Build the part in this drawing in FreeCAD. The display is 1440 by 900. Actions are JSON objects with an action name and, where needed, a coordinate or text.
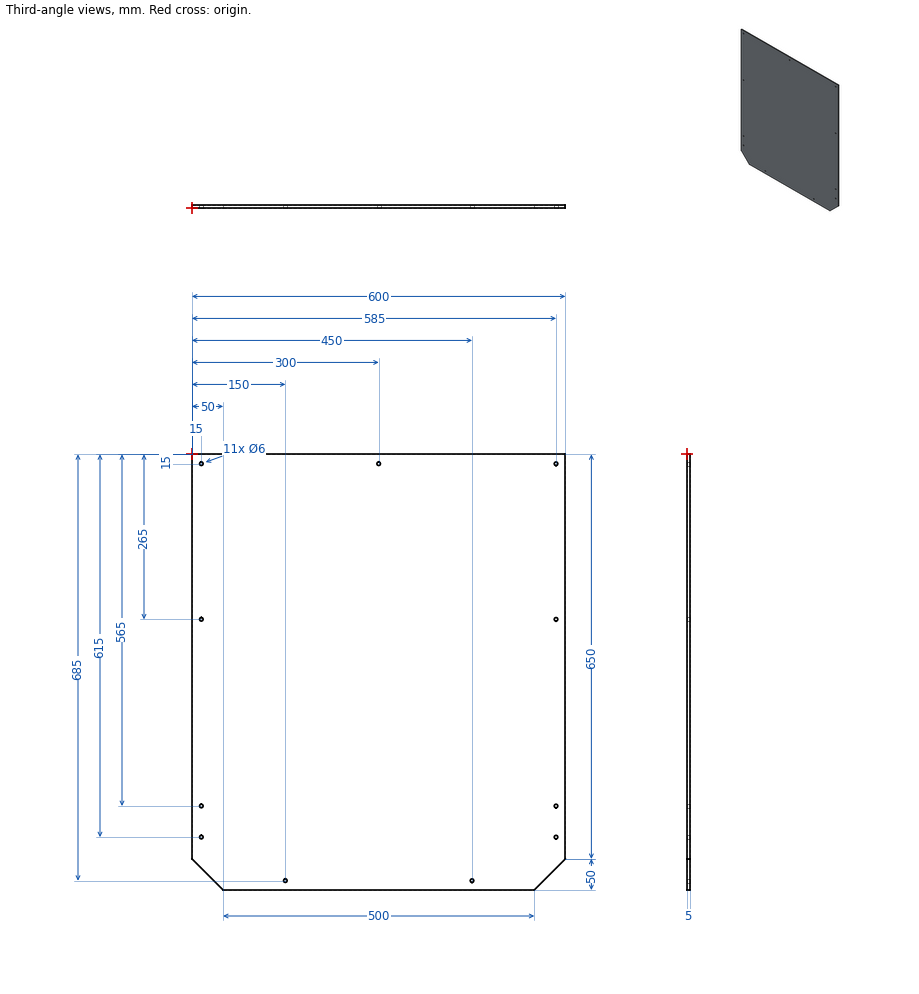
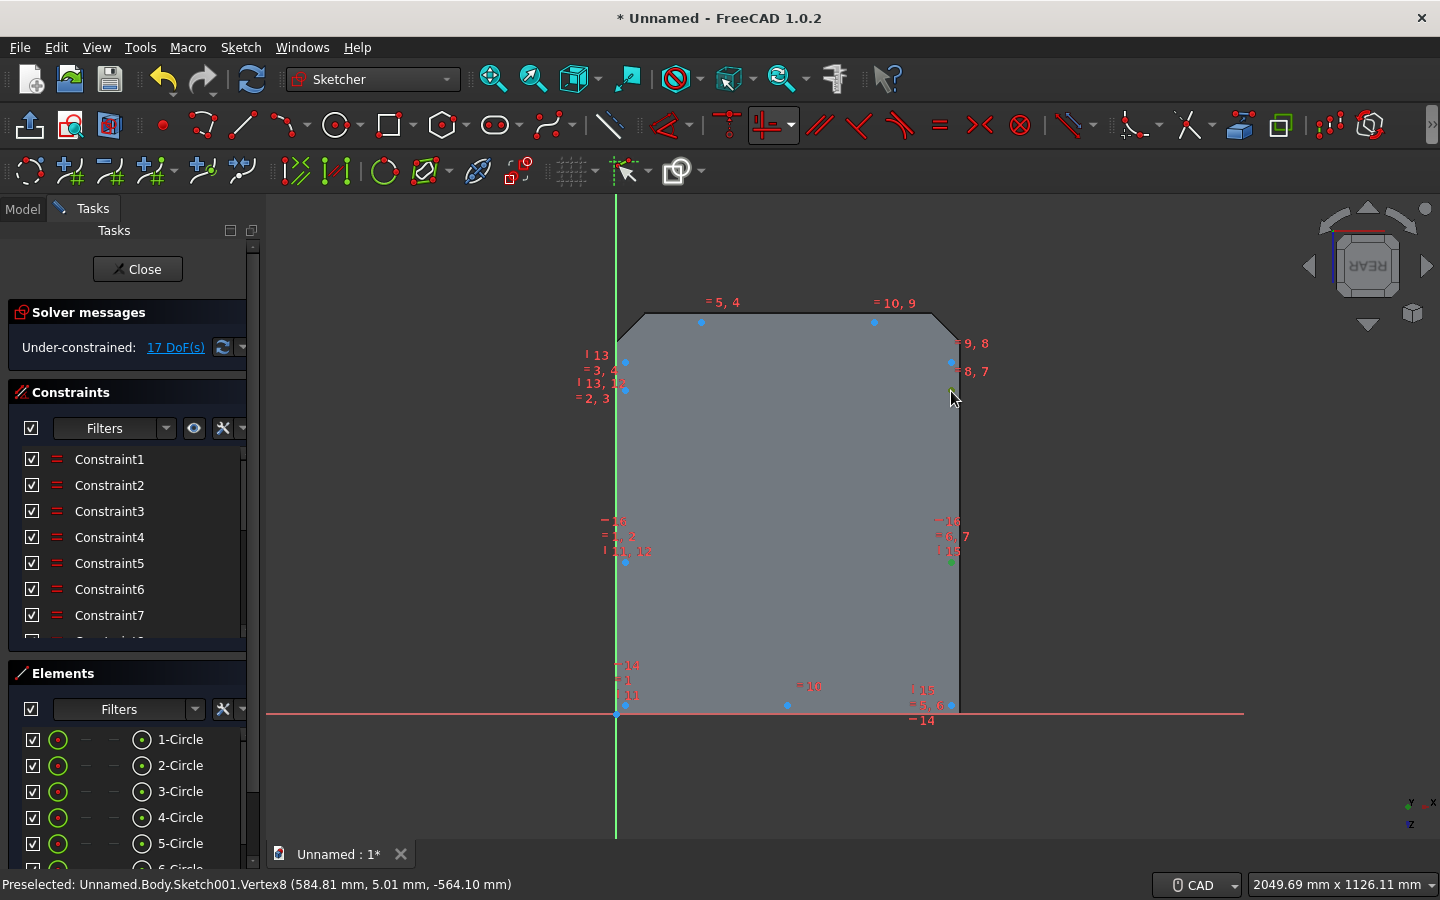
{"action": "key", "text": "v"}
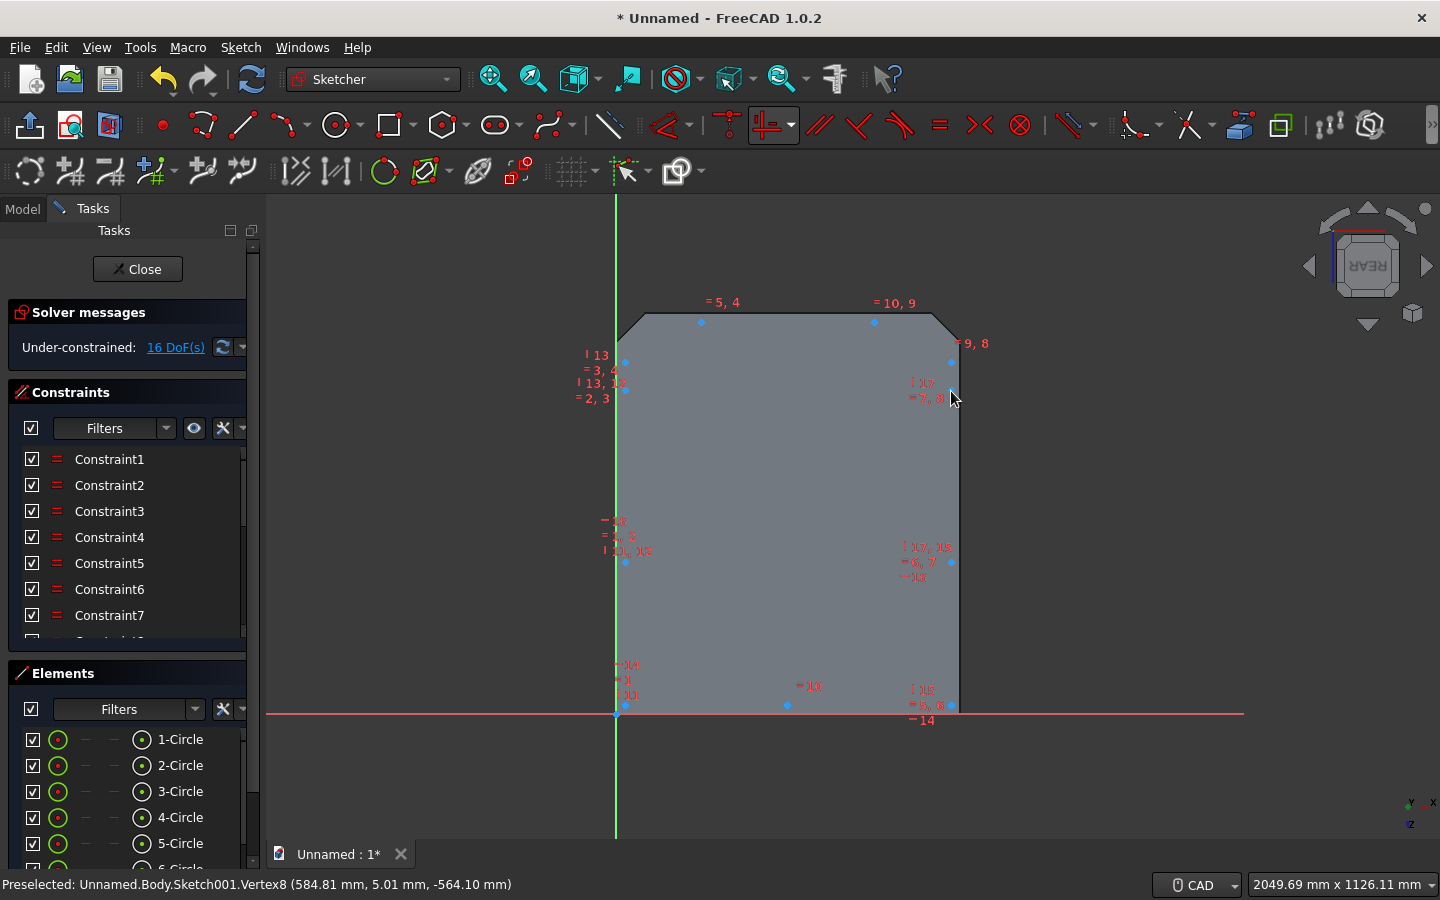
{"action": "left_click", "coordinate": [625, 391]}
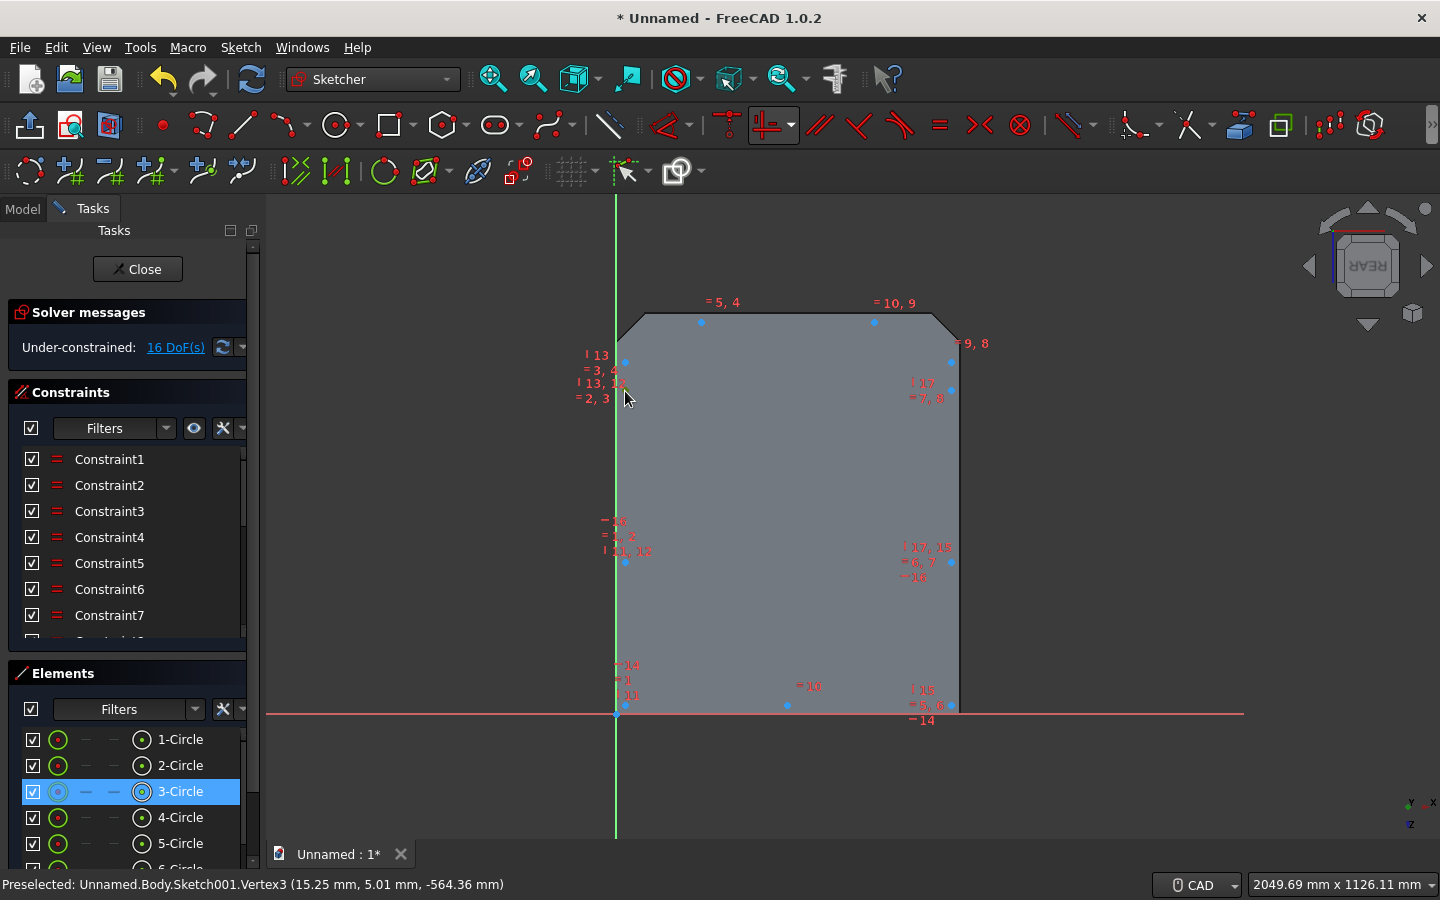
{"action": "left_click", "coordinate": [951, 391]}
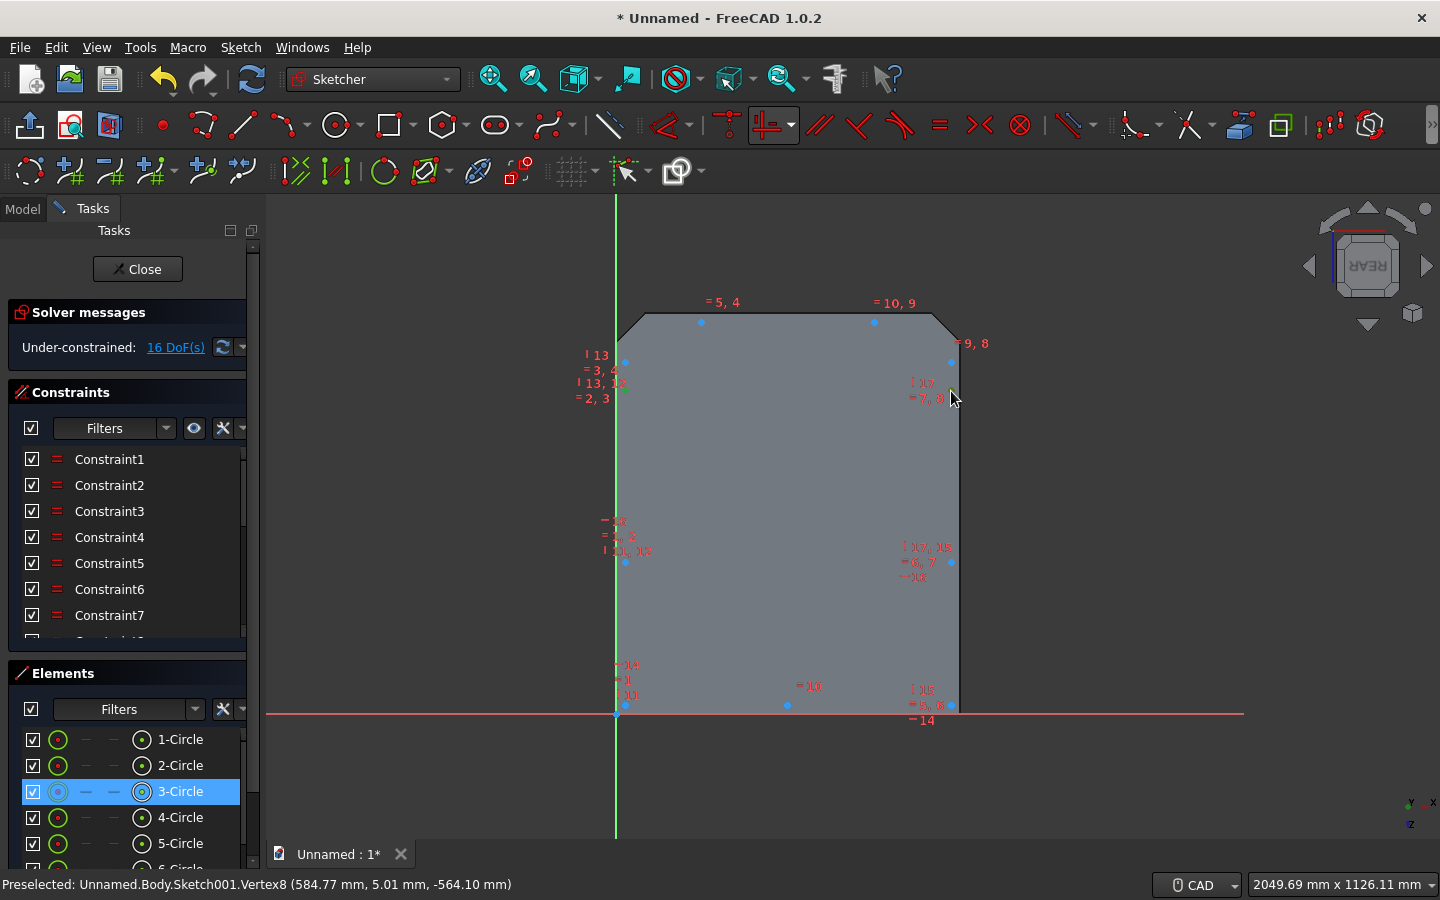
{"action": "key", "text": "h"}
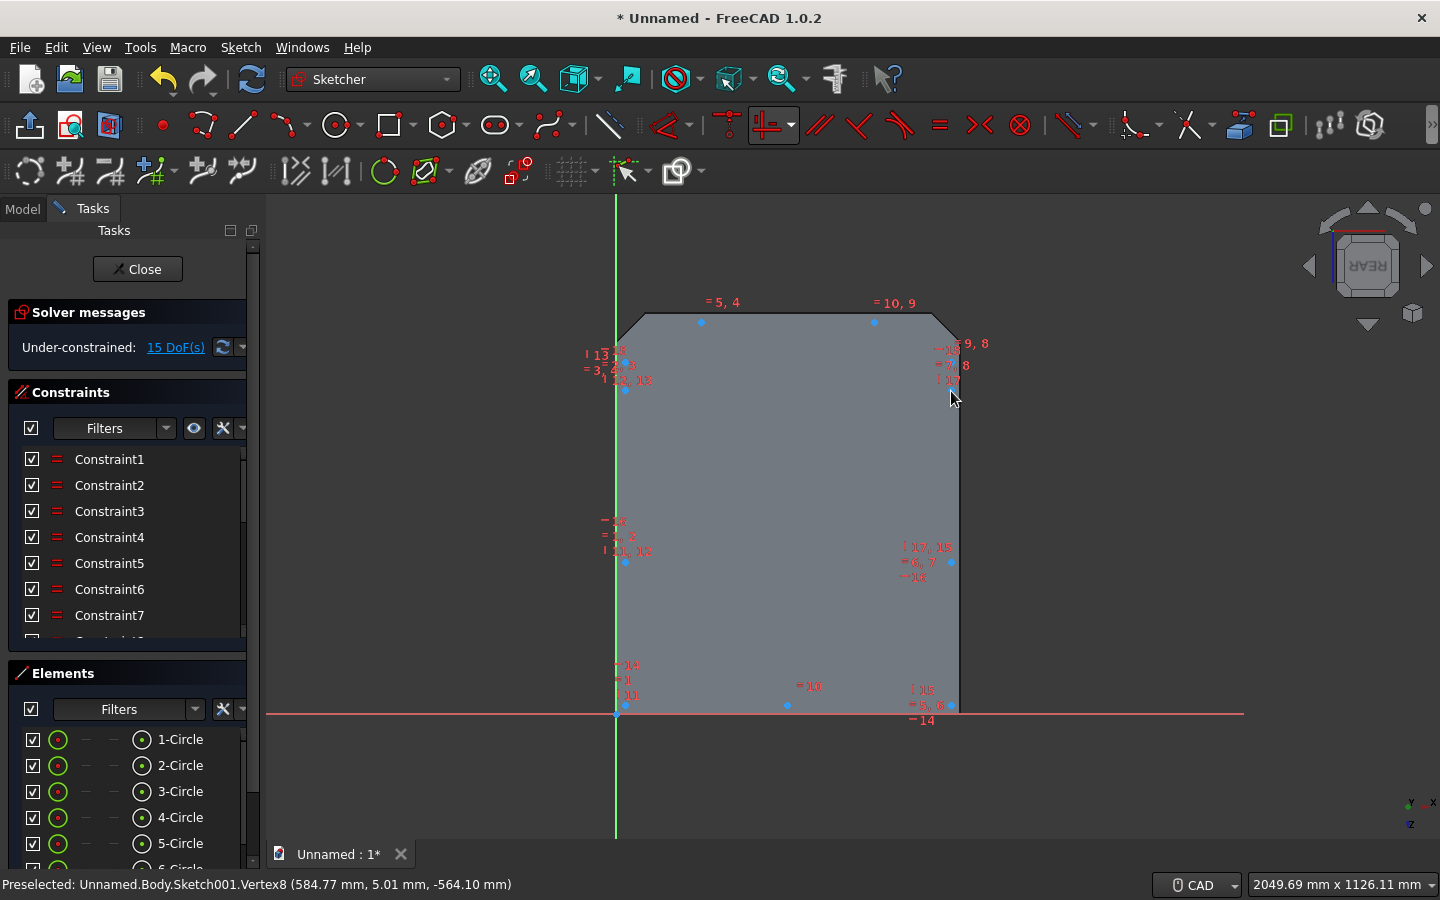
{"action": "left_click", "coordinate": [951, 391]}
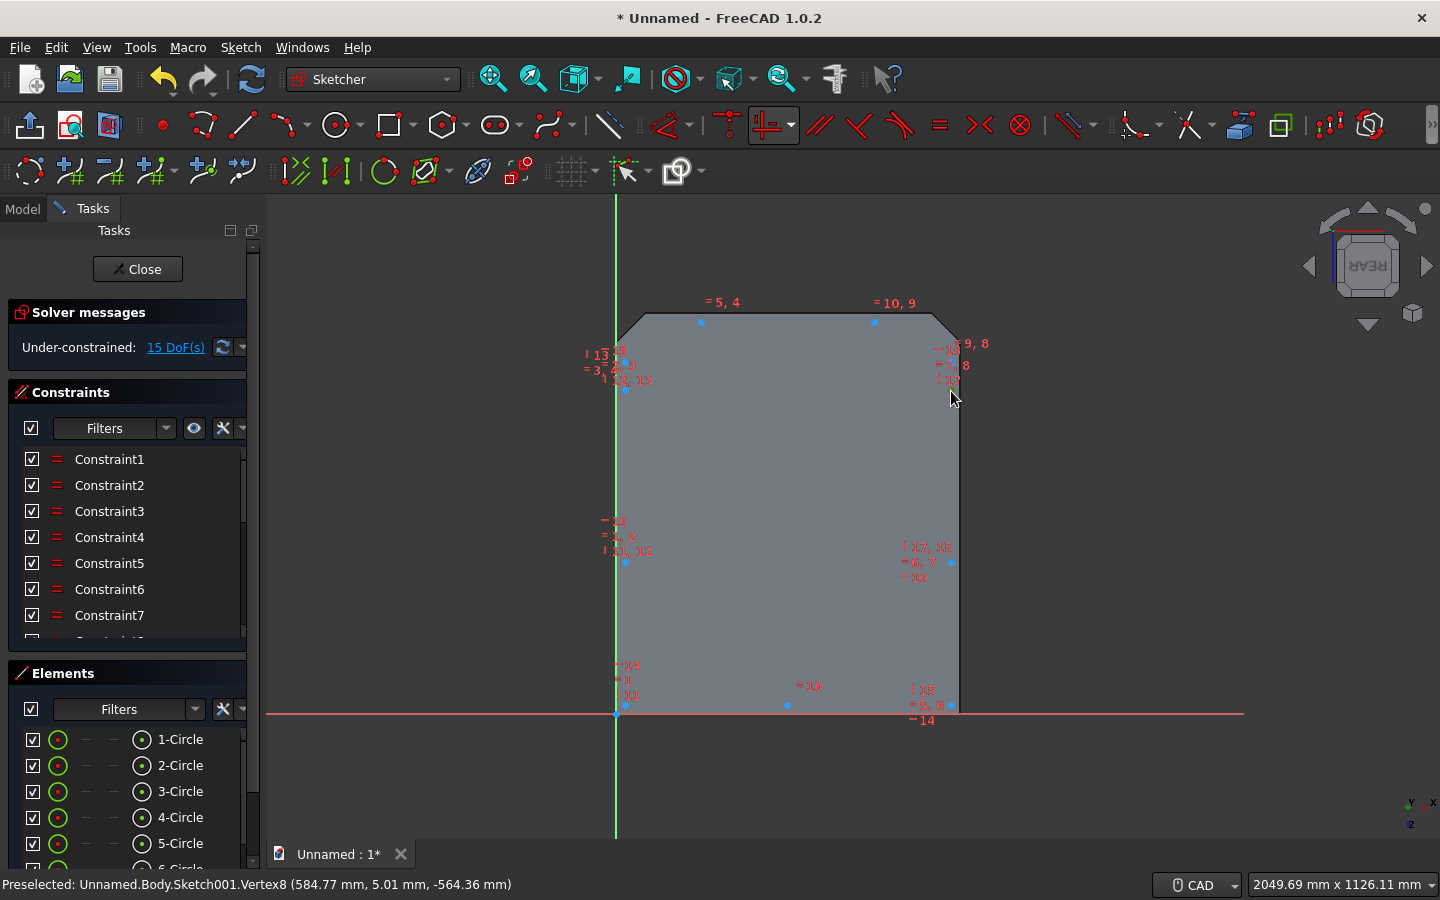
{"action": "scroll", "coordinate": [951, 363], "scroll_direction": "up", "scroll_amount": 4}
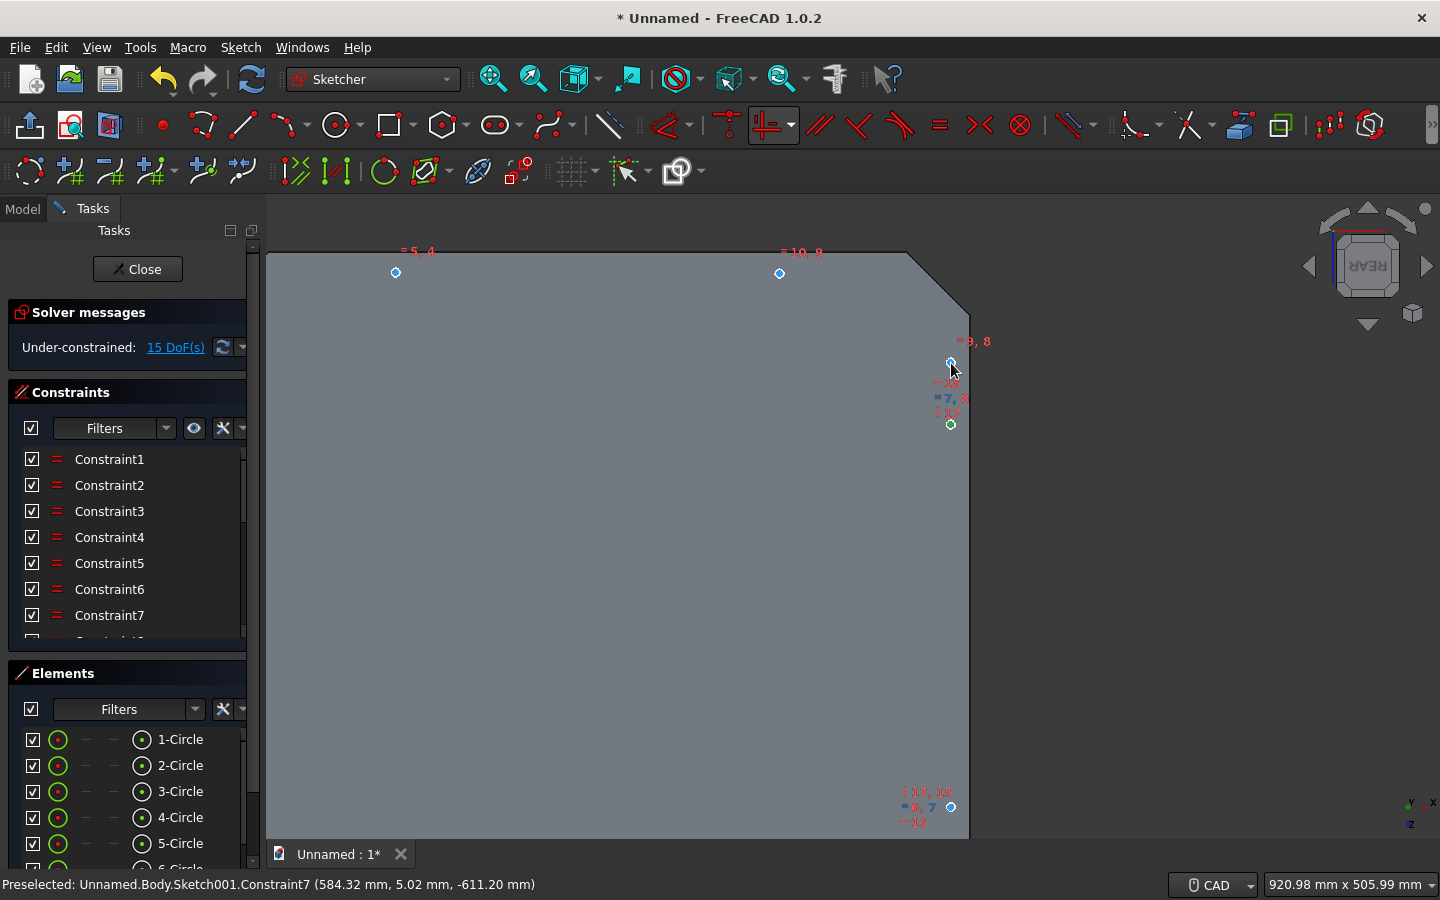
{"action": "left_click", "coordinate": [951, 363]}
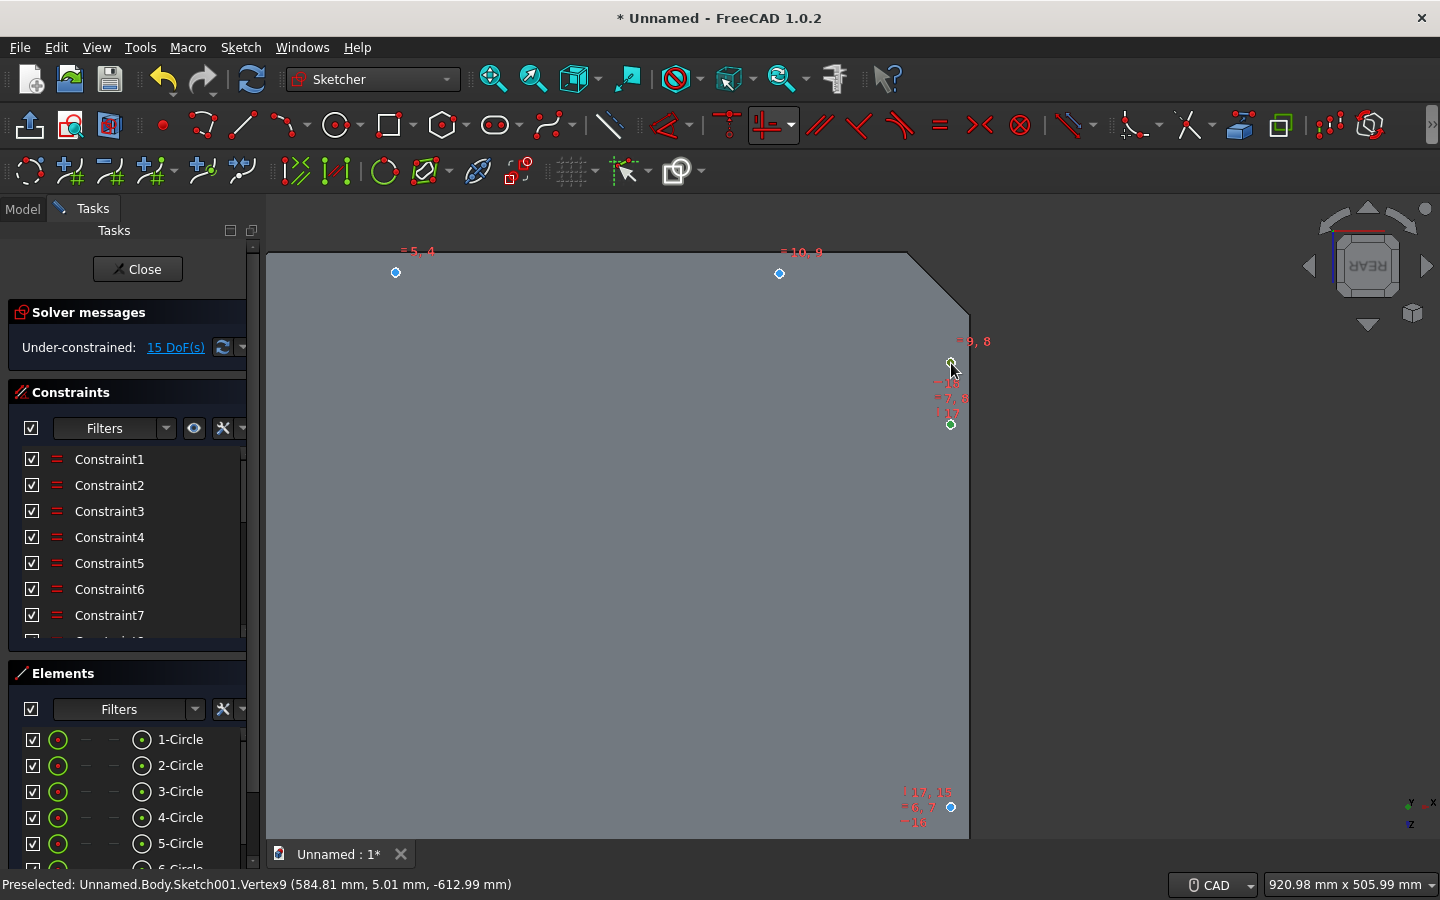
{"action": "key", "text": "v"}